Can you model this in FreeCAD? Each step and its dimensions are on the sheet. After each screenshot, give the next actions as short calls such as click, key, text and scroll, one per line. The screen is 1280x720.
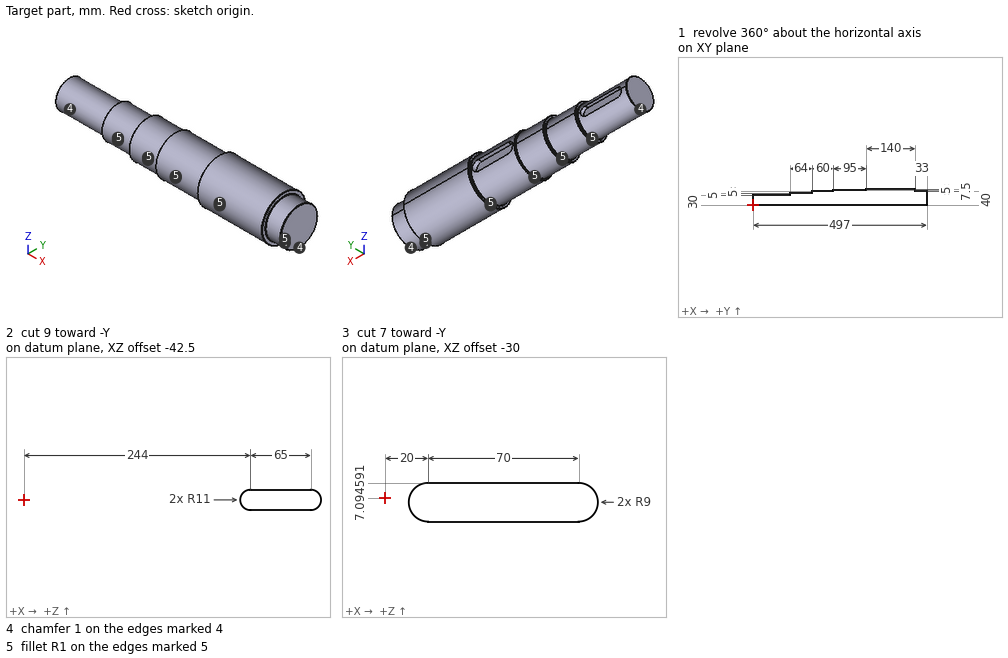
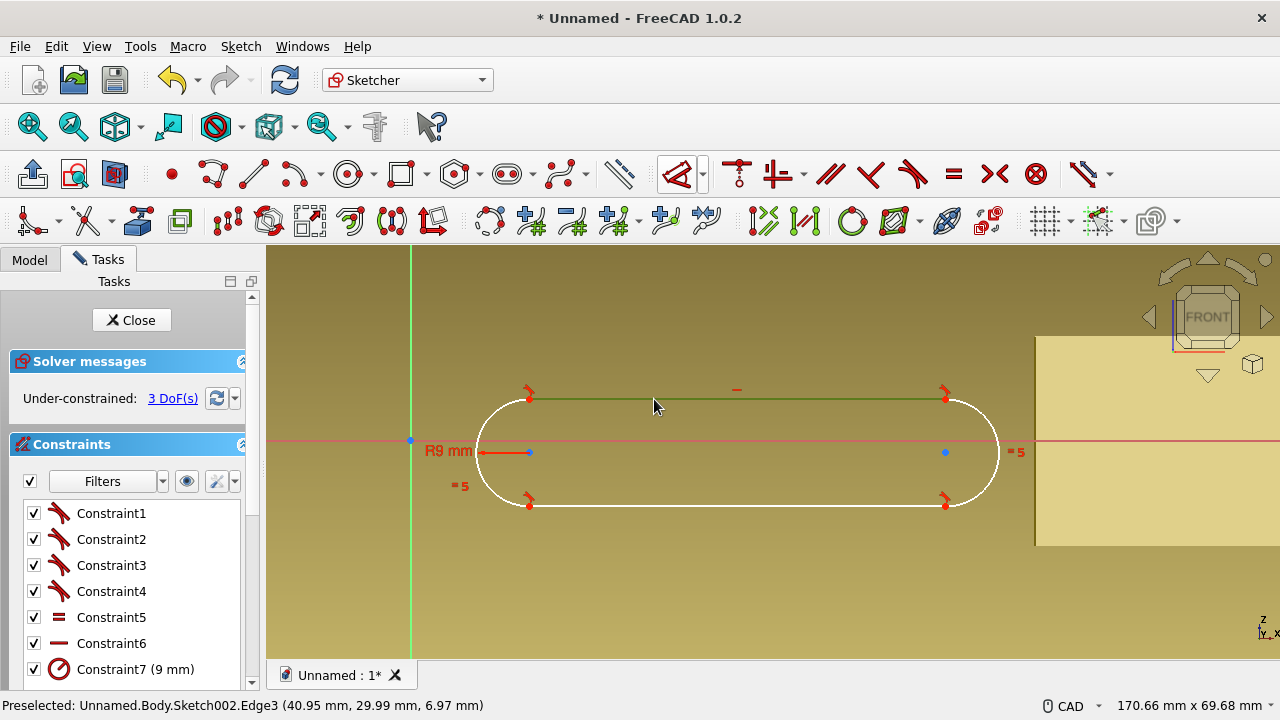
key(l)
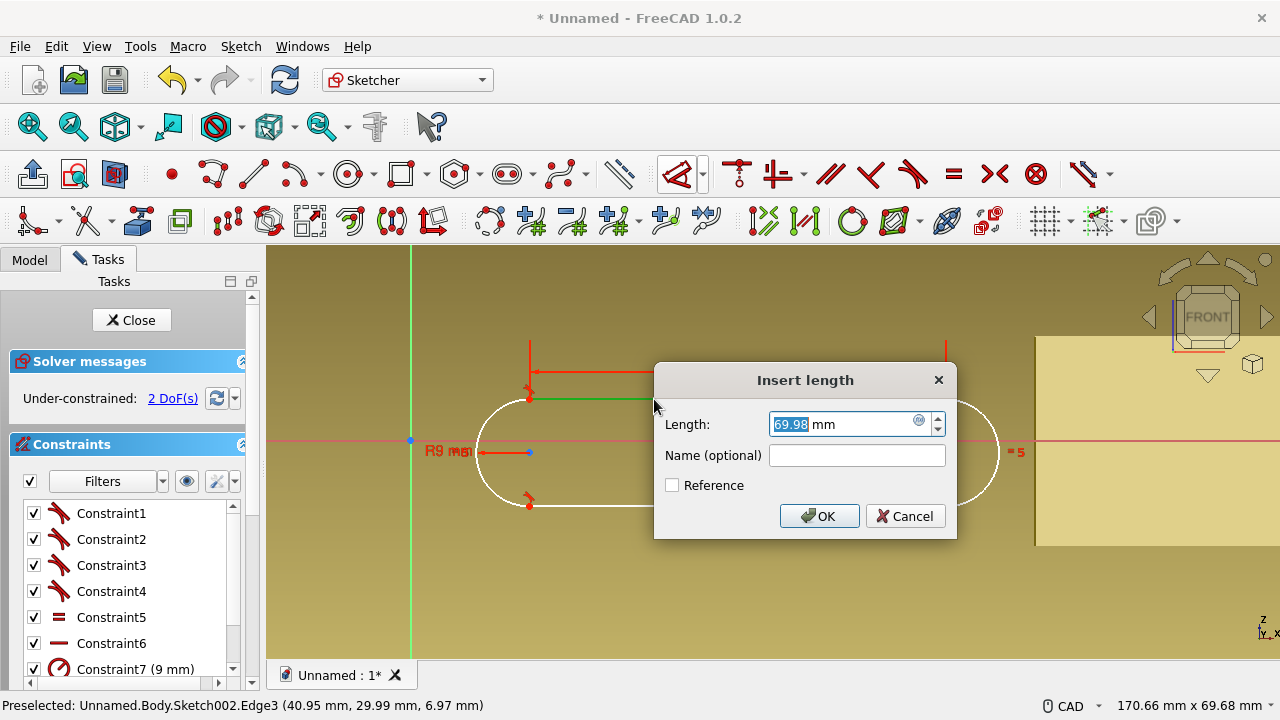
text(70)
key(Return)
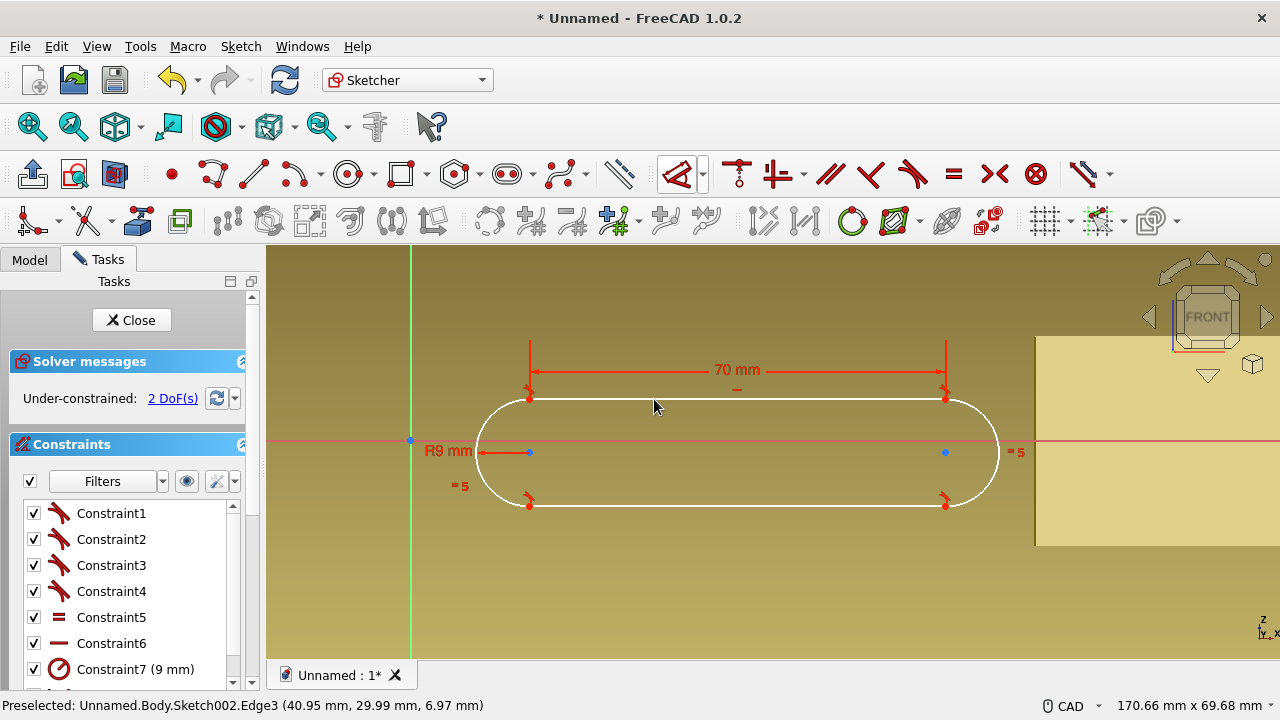
click(530, 399)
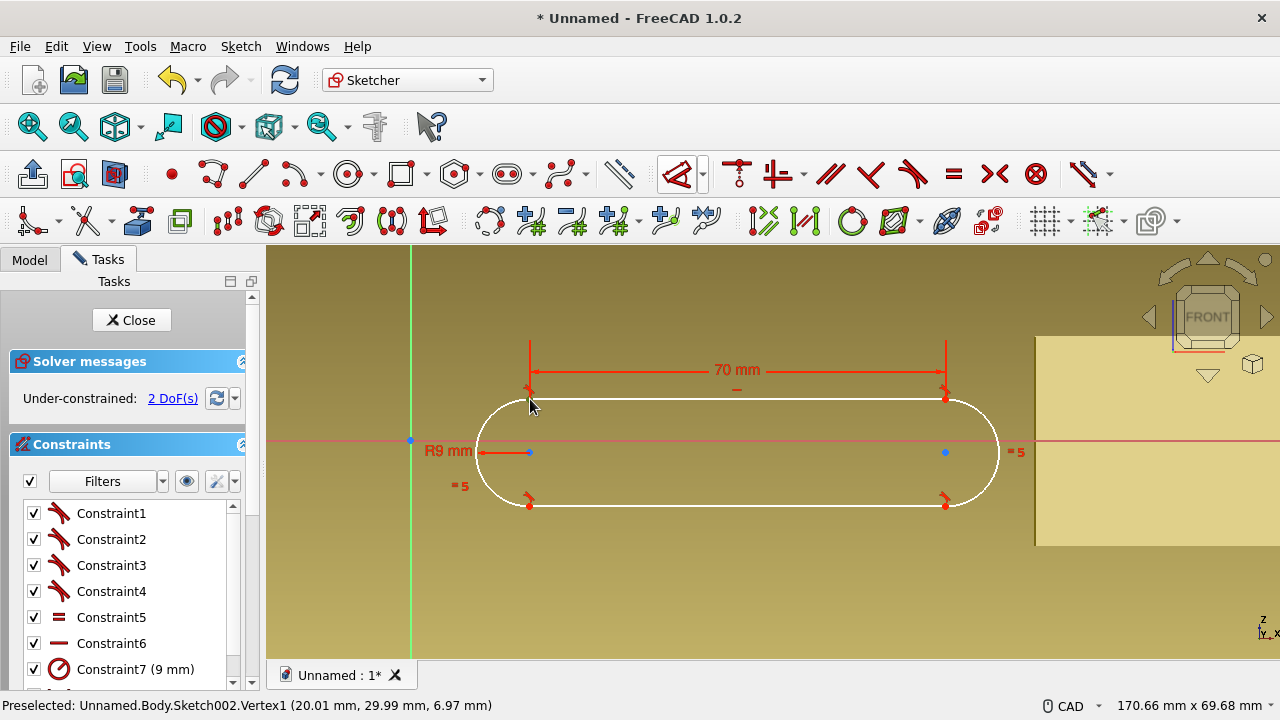
key(l)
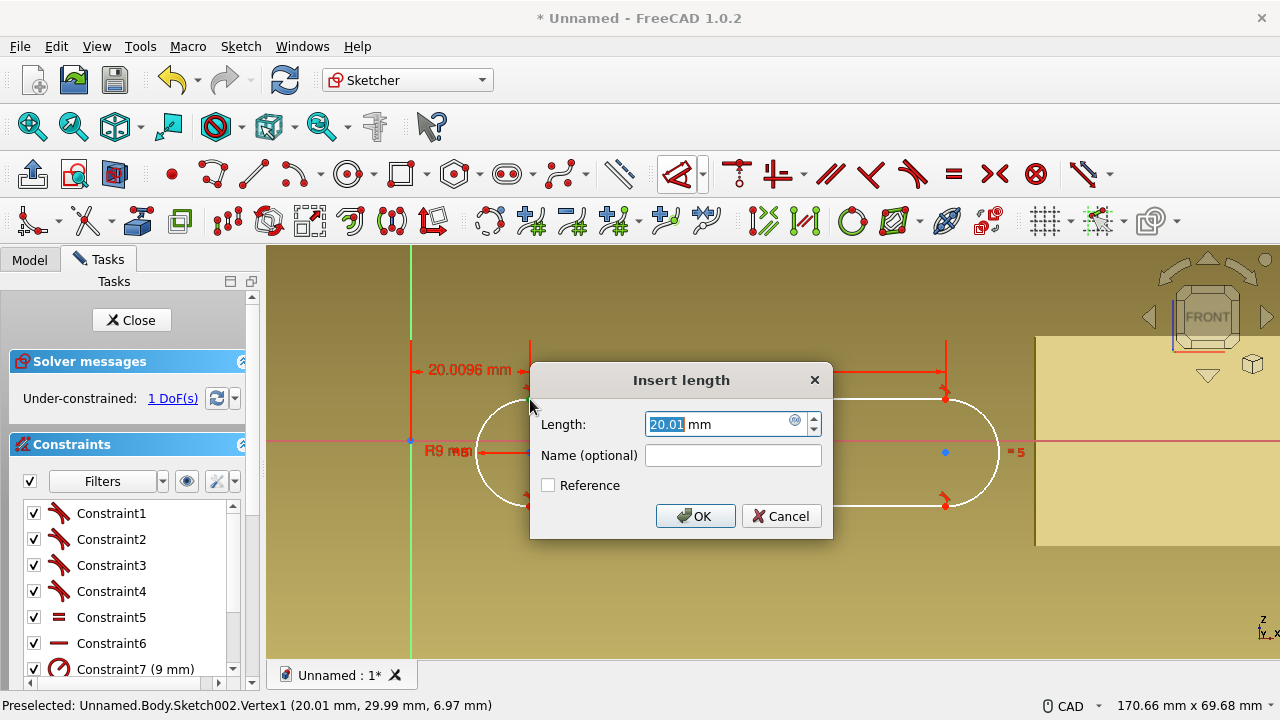
text(20)
key(Return)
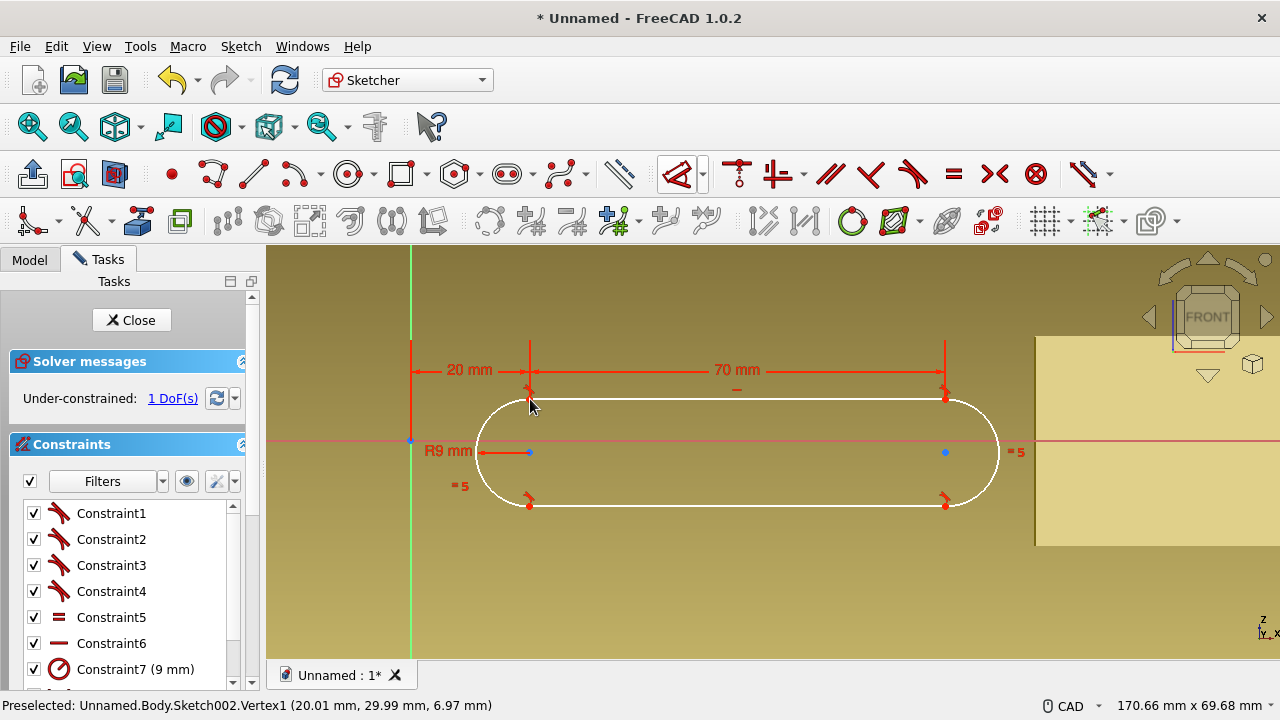
click(530, 399)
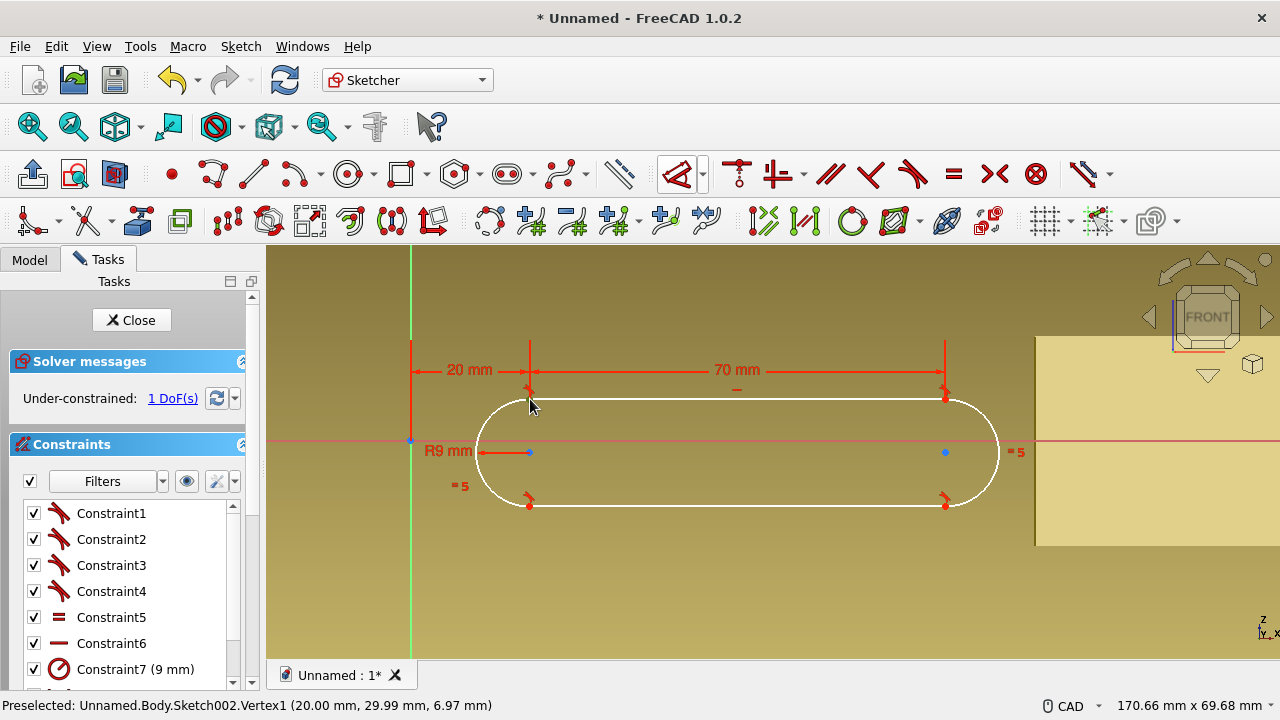
click(702, 174)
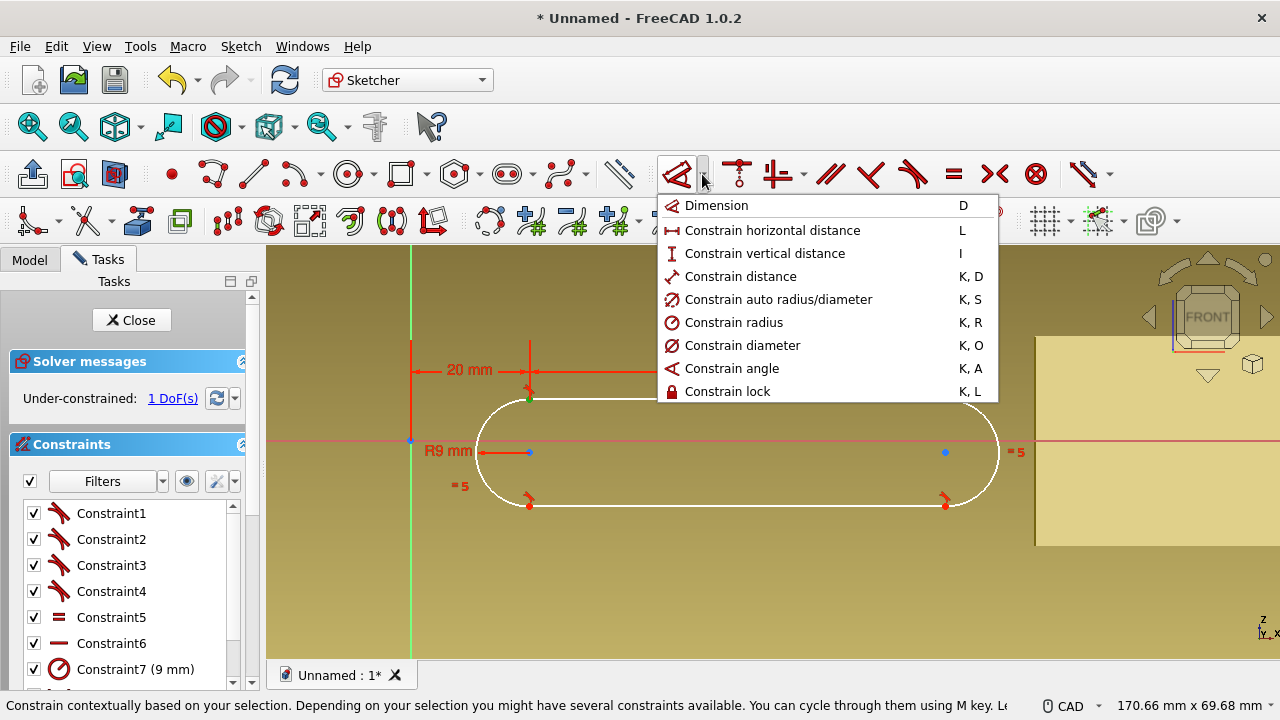
click(828, 254)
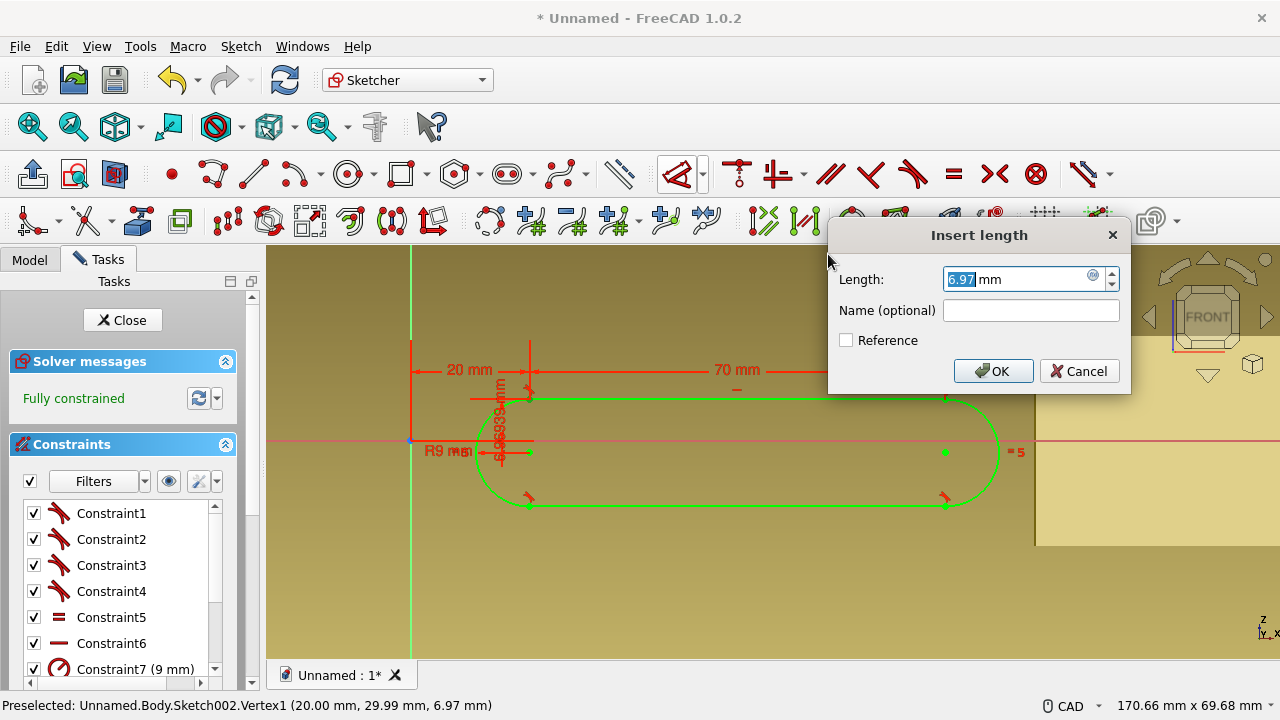
text(7.094591)
key(Return)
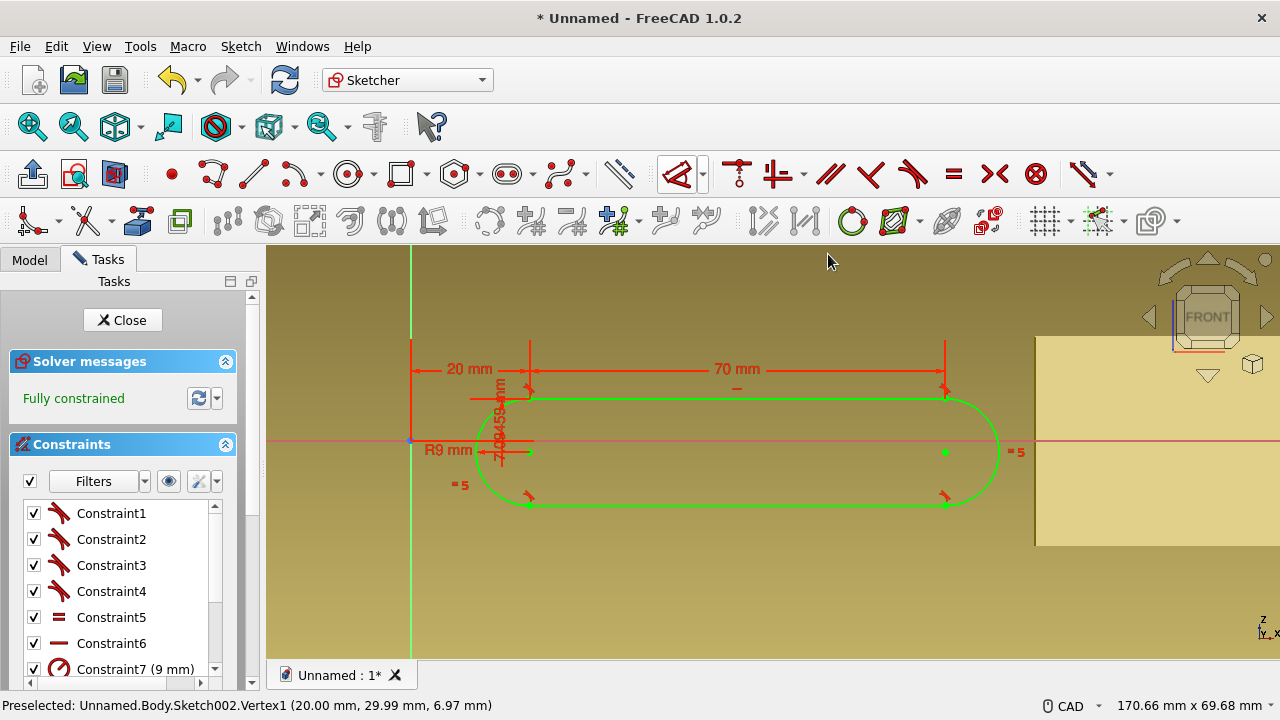
click(123, 320)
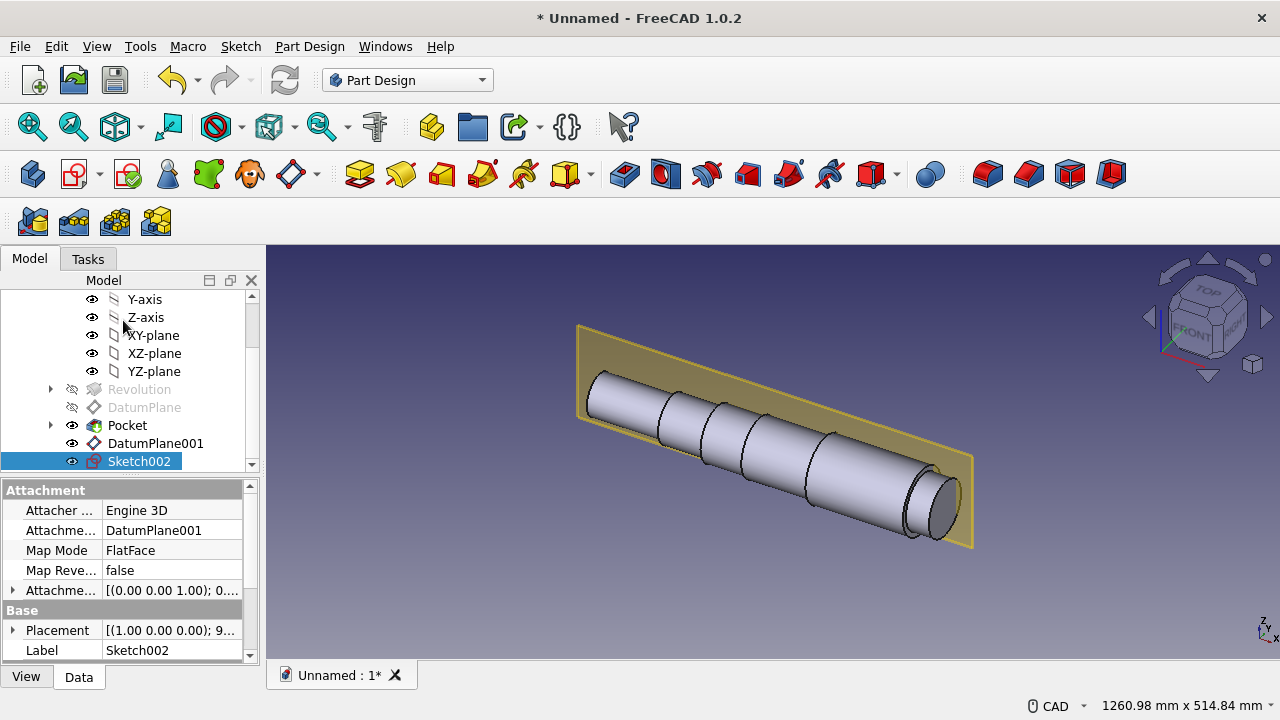
click(625, 174)